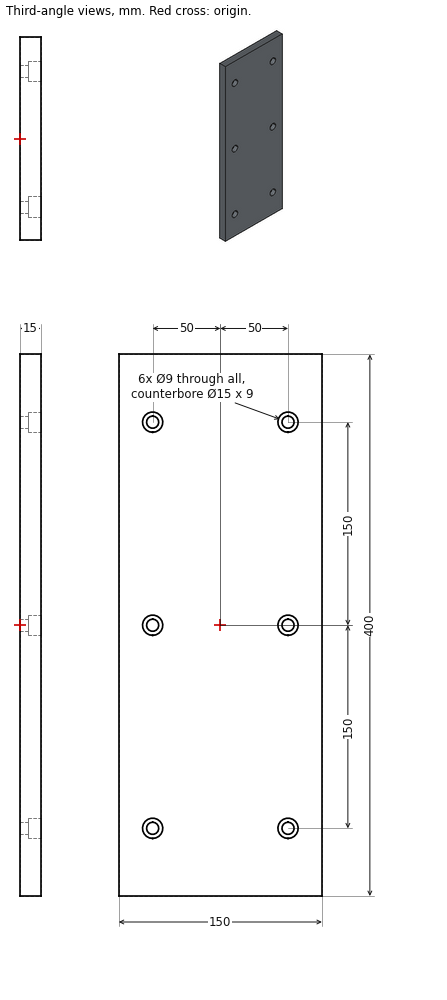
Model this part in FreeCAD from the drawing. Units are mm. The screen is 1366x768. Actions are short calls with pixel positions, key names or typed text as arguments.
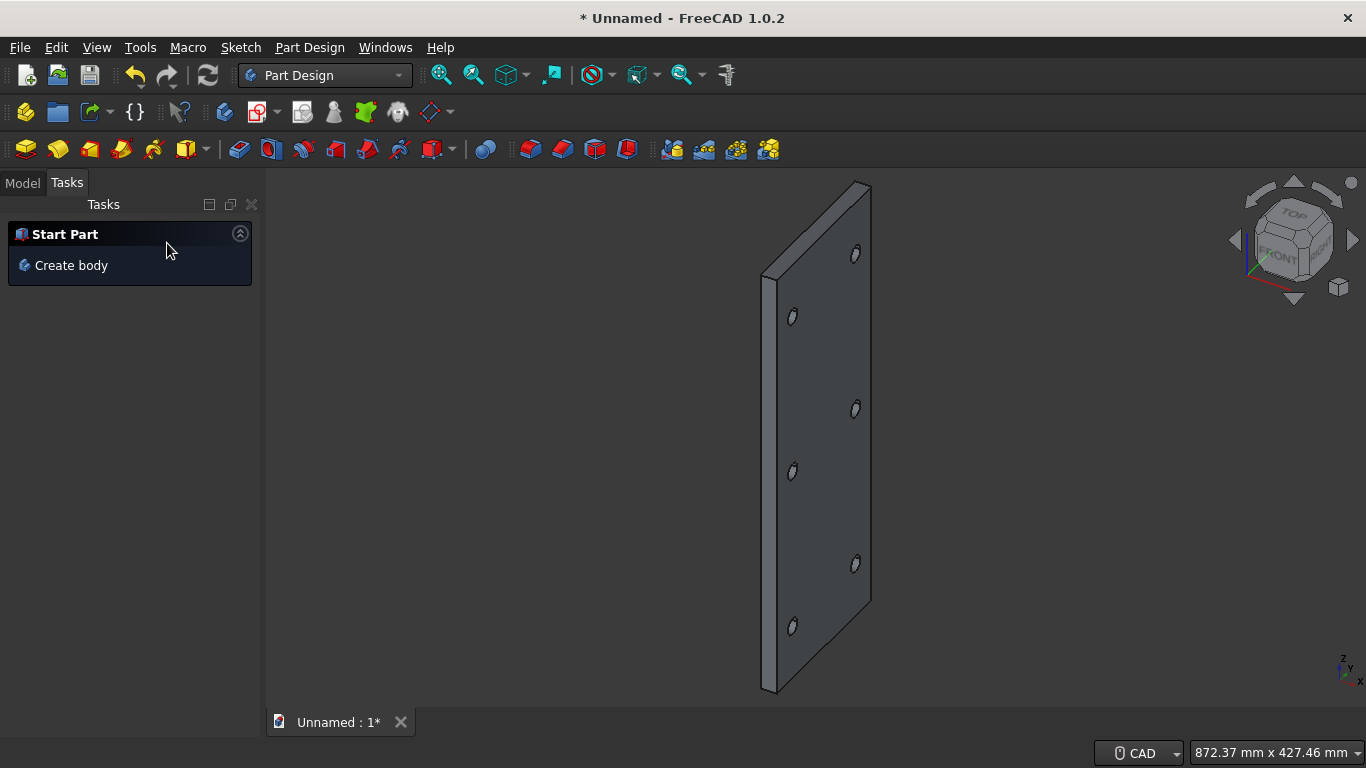
key(0)